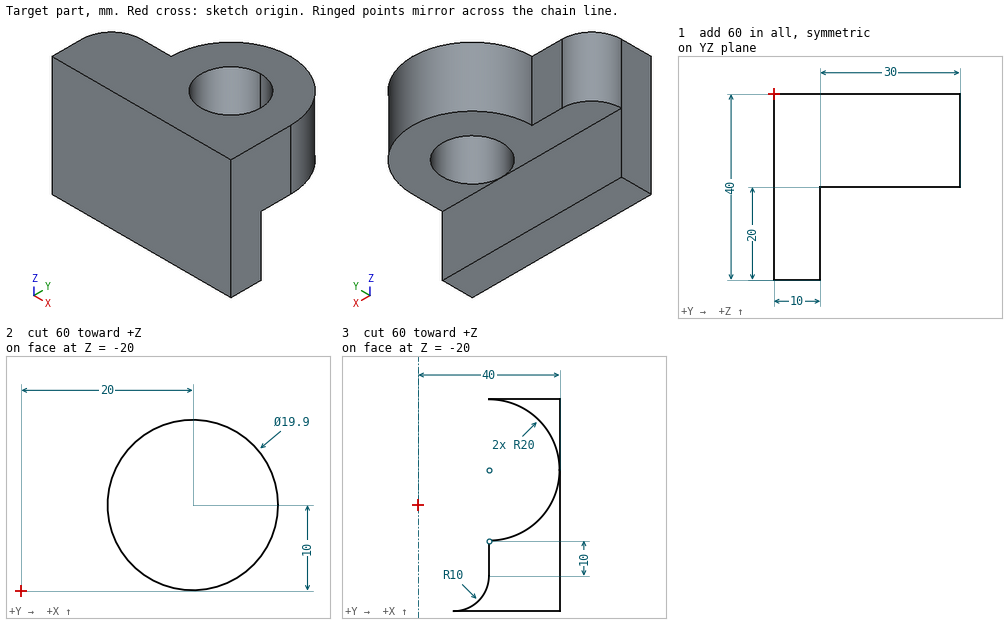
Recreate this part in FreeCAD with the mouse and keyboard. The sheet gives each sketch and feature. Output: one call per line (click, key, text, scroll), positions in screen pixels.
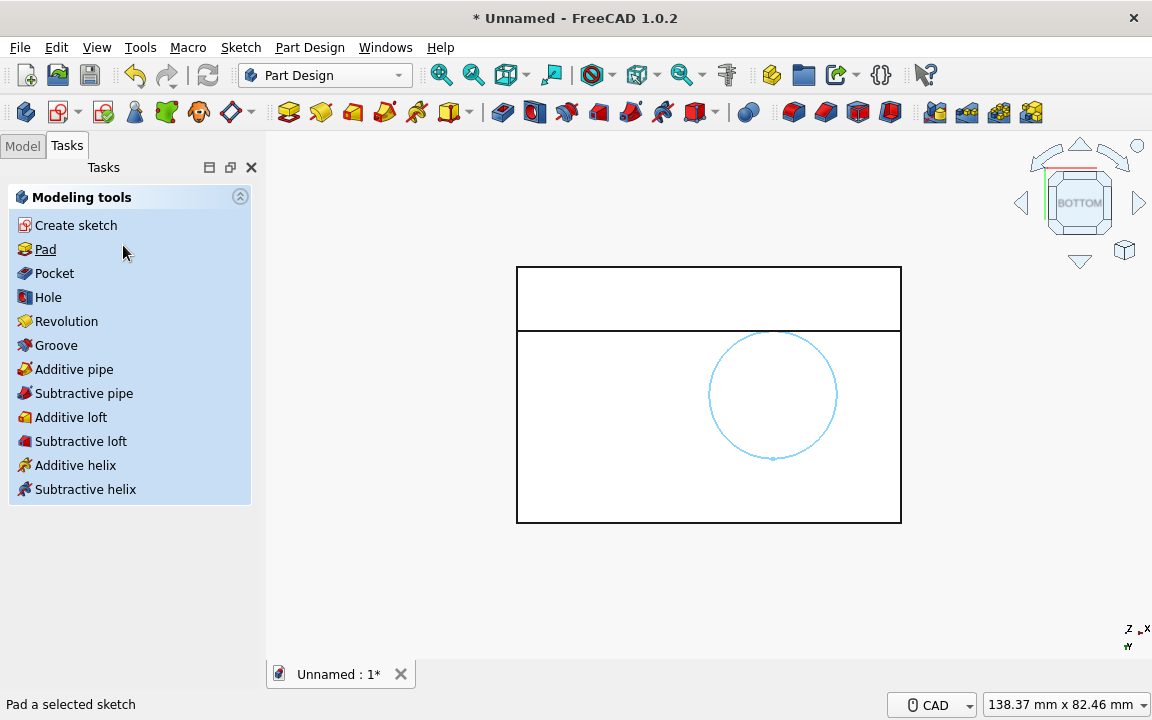
click(504, 112)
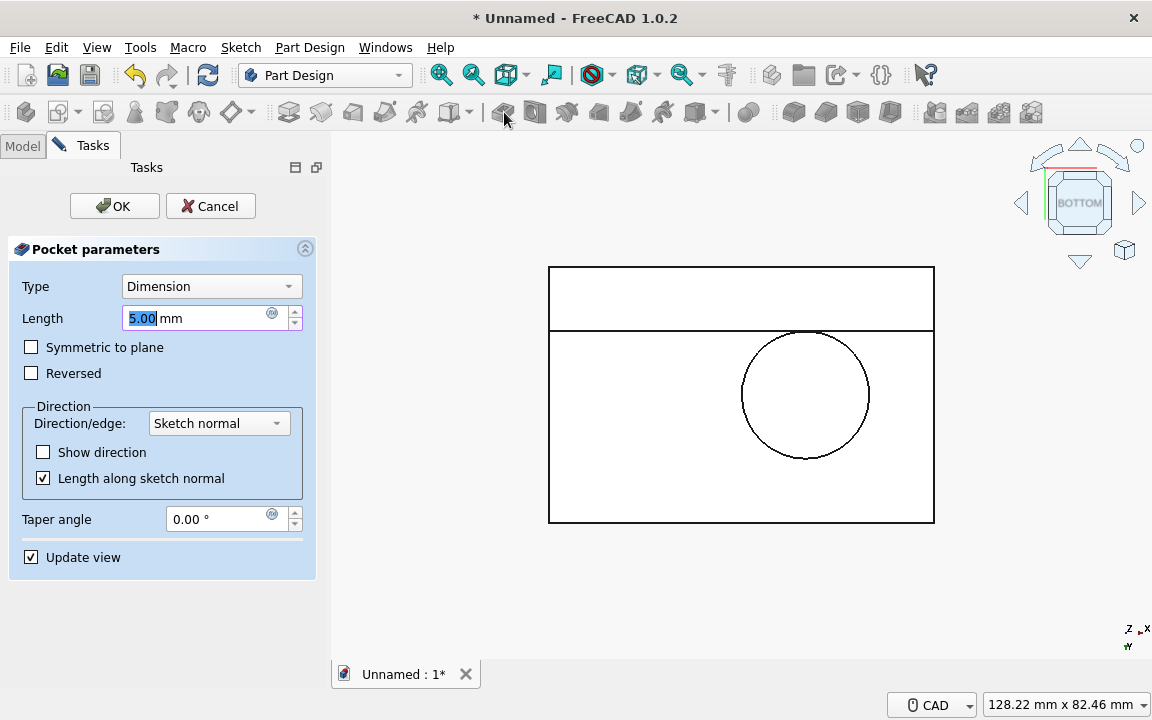
text(60)
key(Tab)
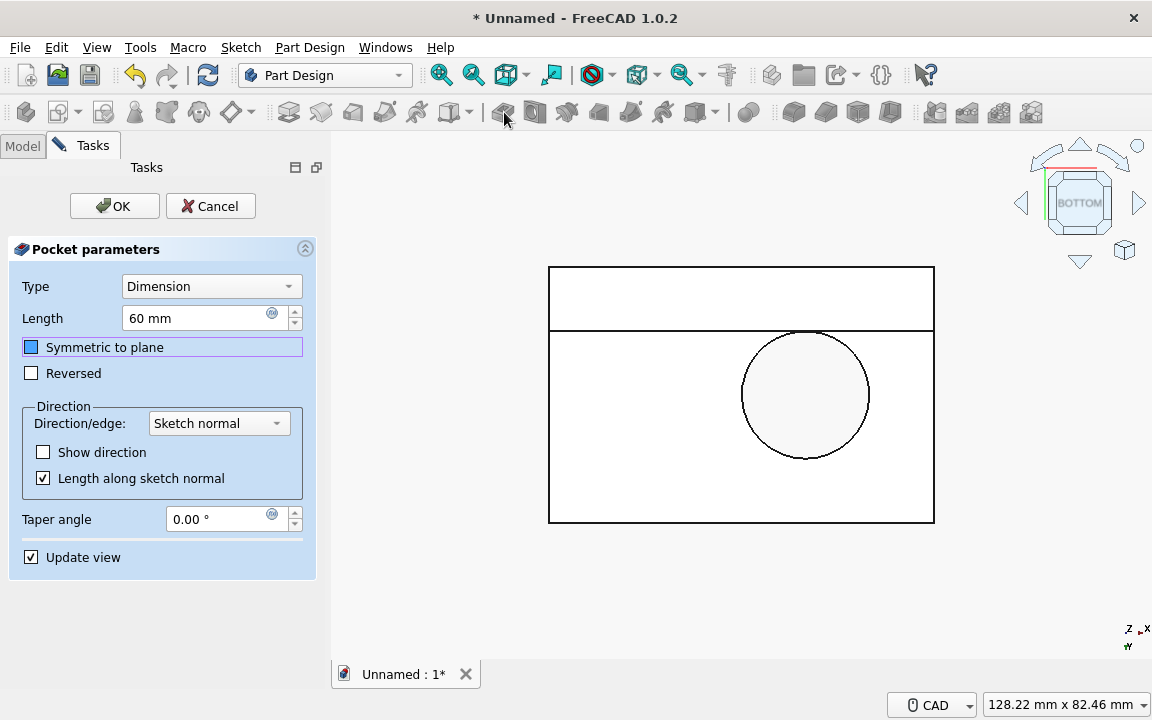
click(115, 206)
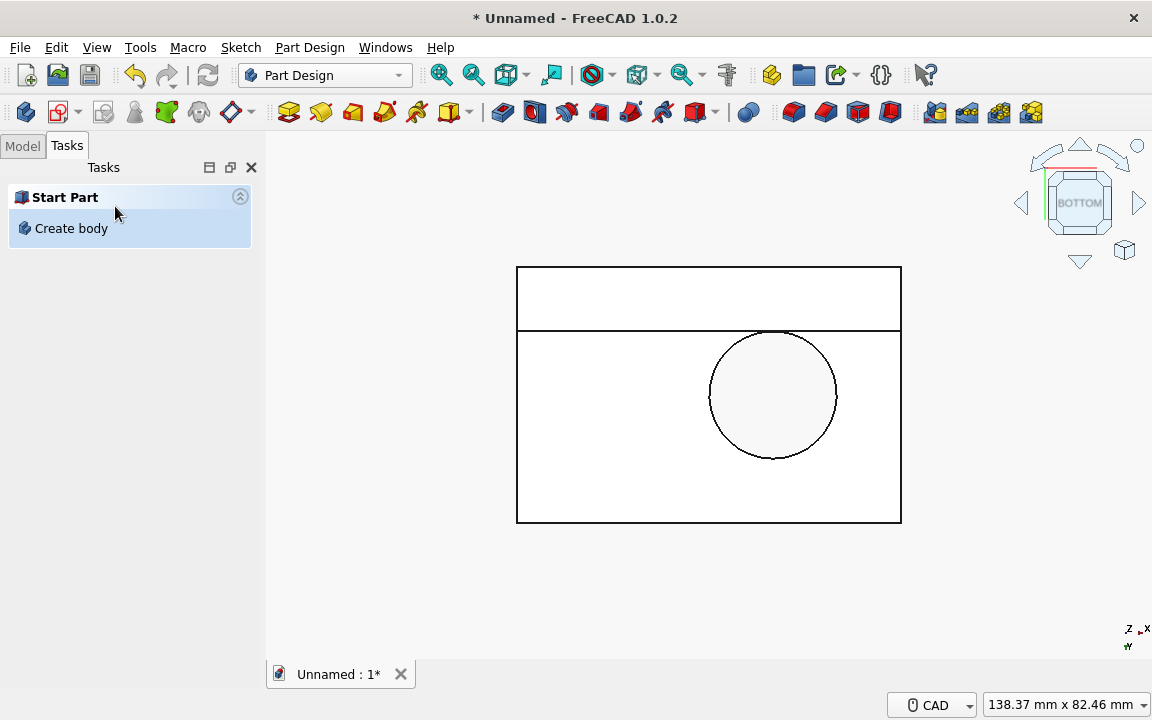
click(599, 426)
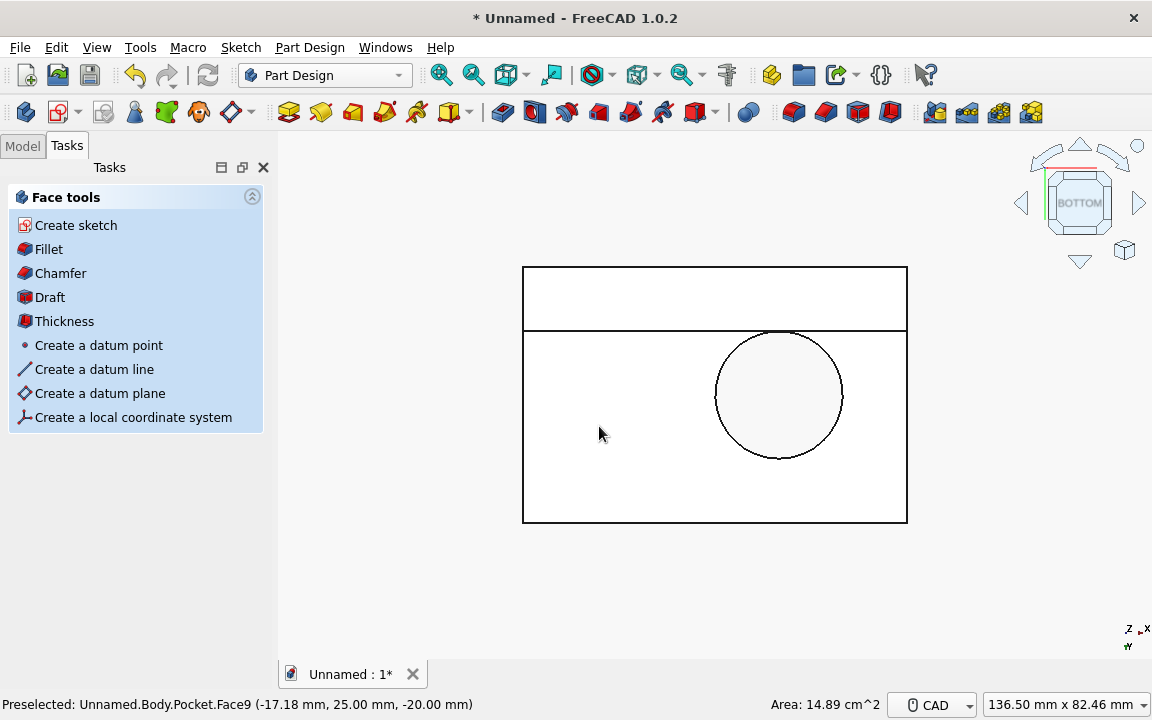
click(58, 112)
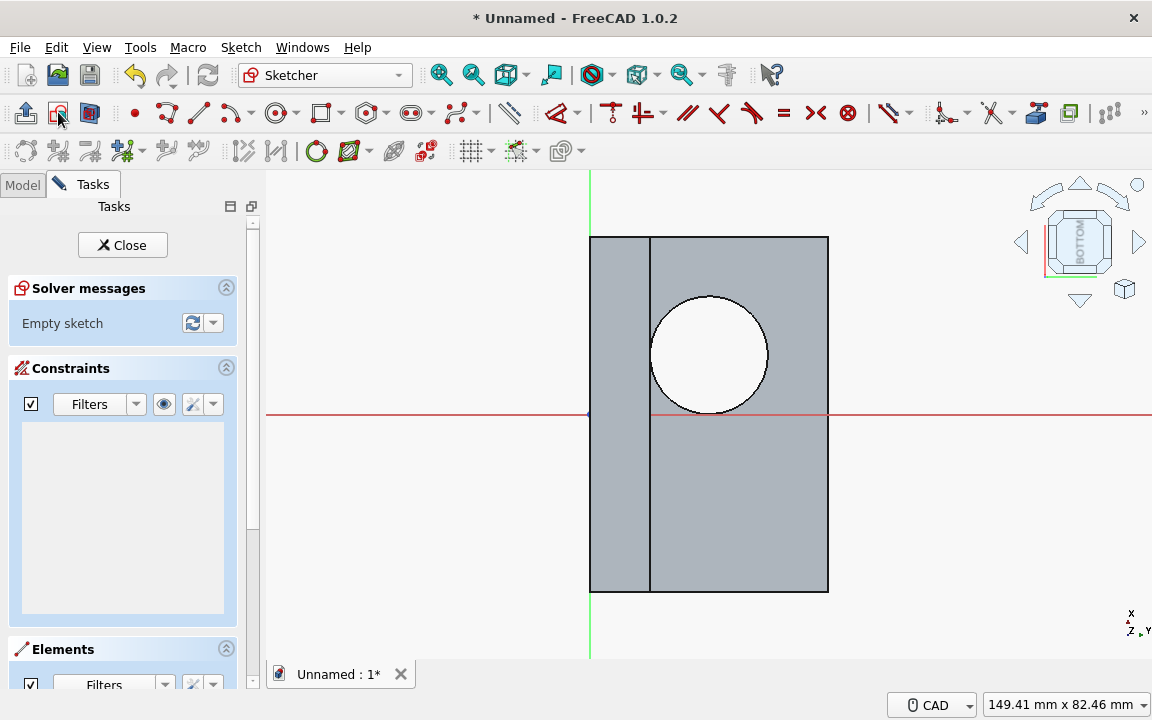
click(90, 114)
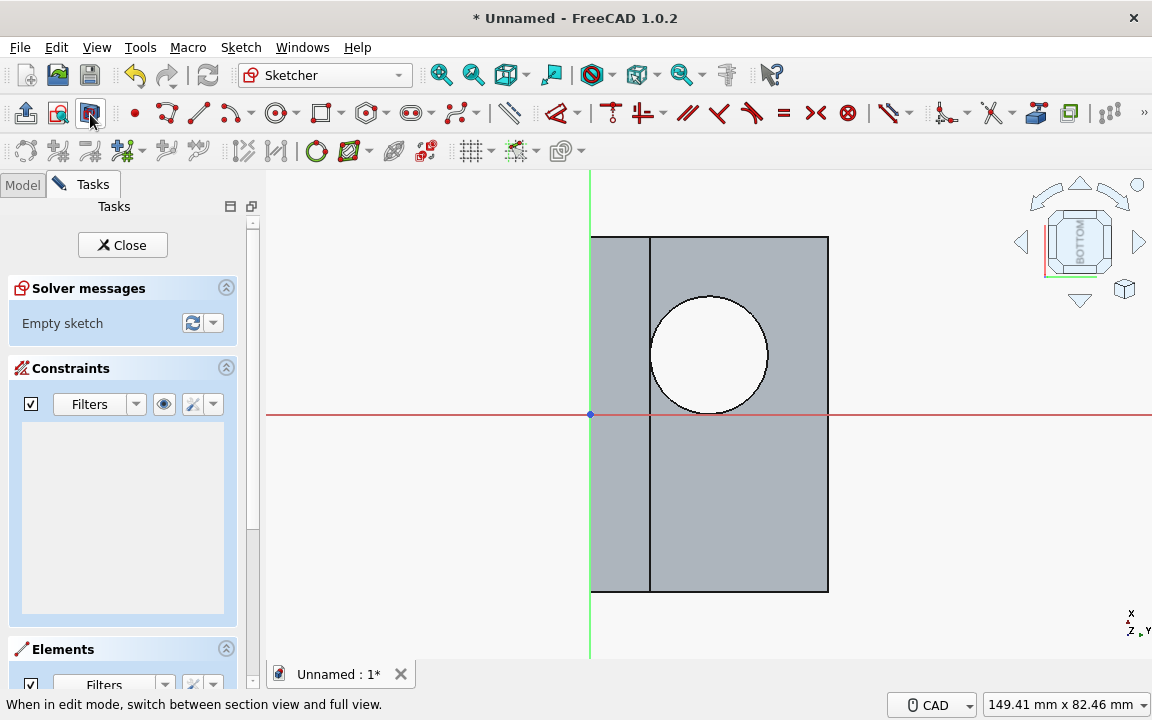
click(168, 114)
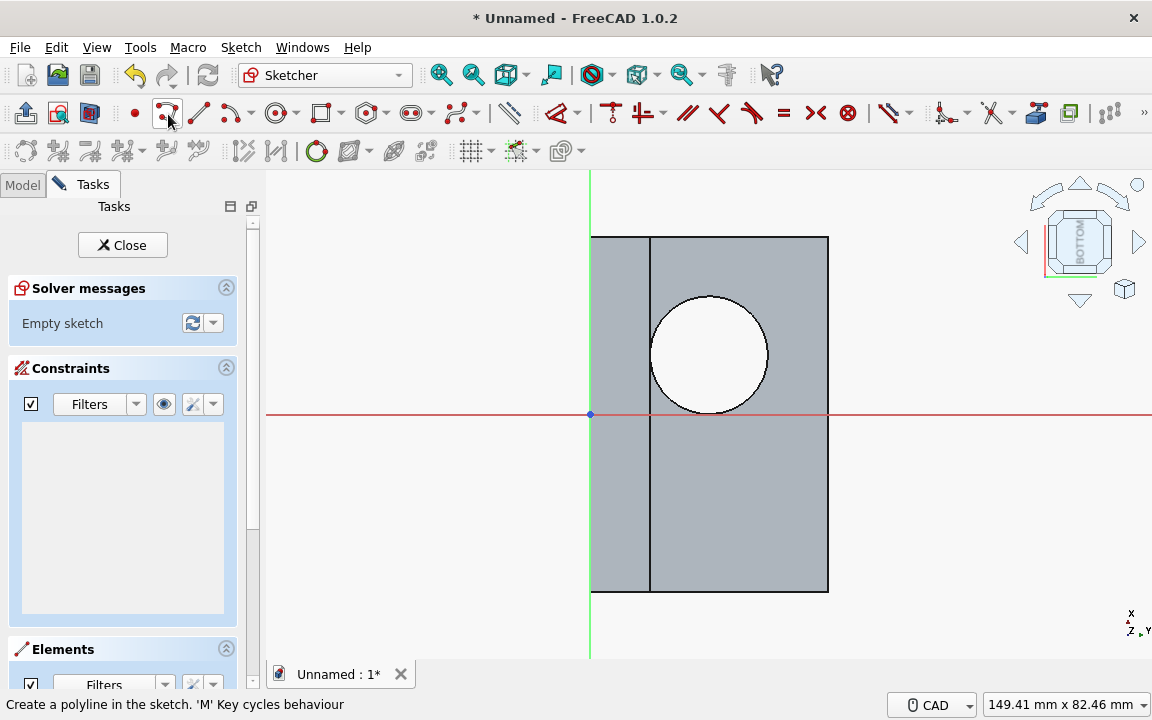
click(828, 355)
click(828, 237)
click(709, 237)
right_click(709, 237)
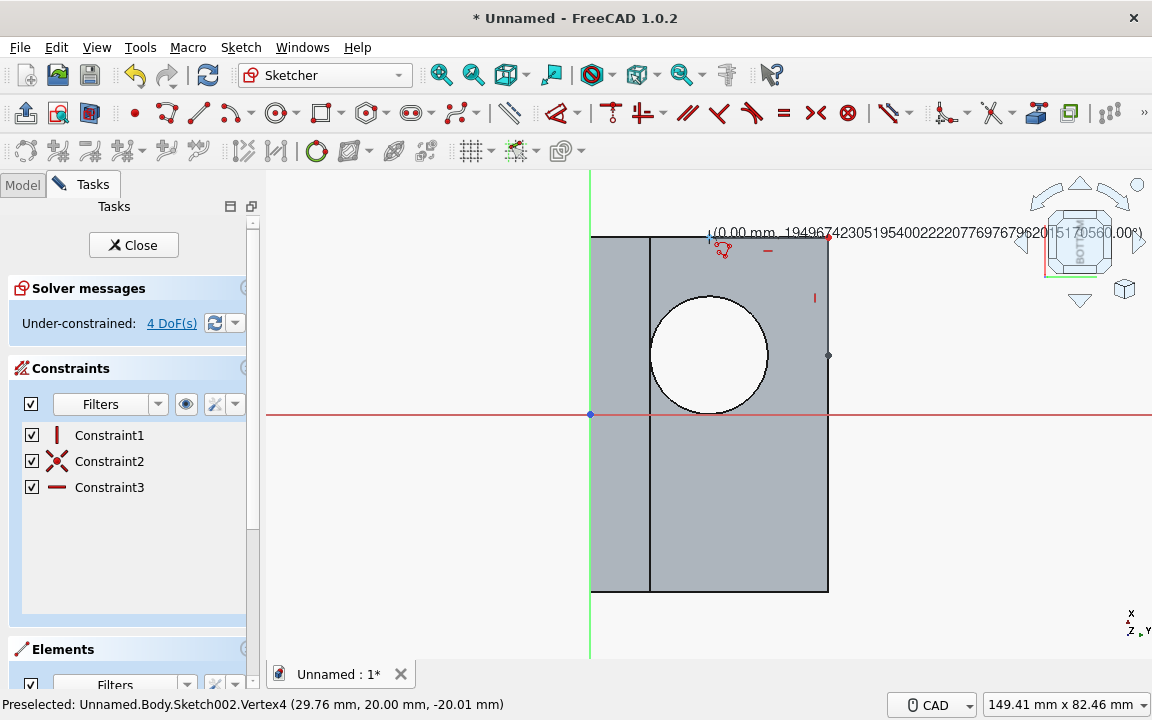
click(254, 114)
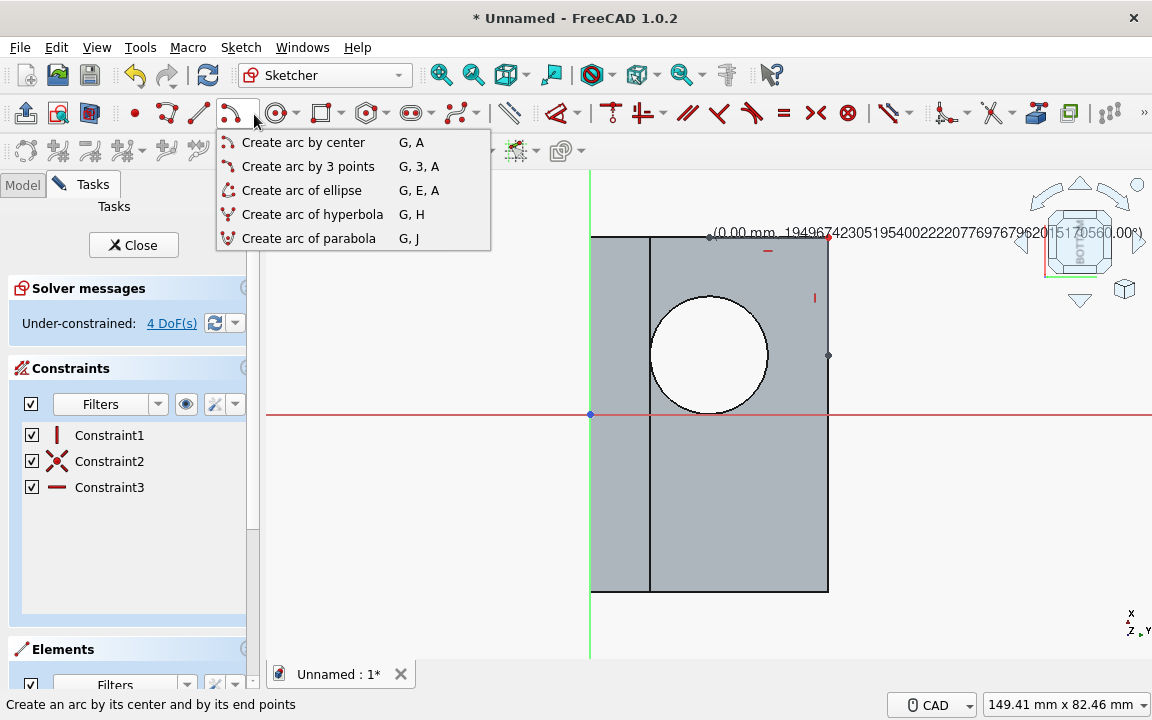
click(354, 166)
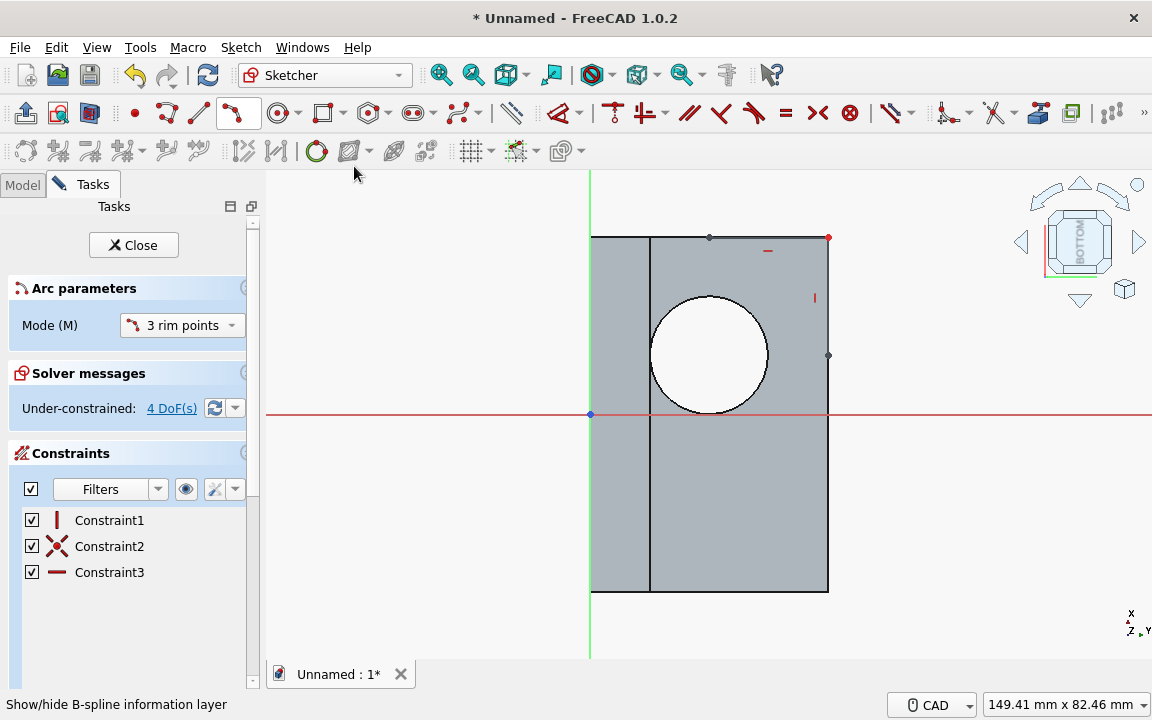
click(709, 238)
click(828, 356)
click(793, 271)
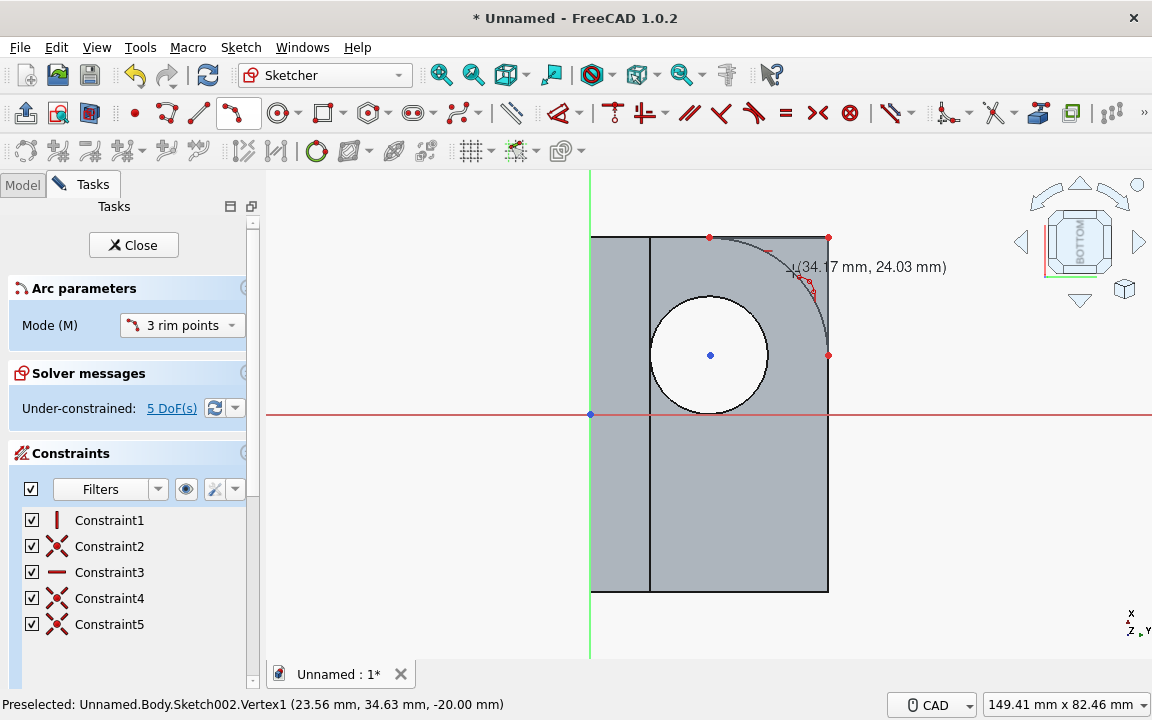
click(200, 114)